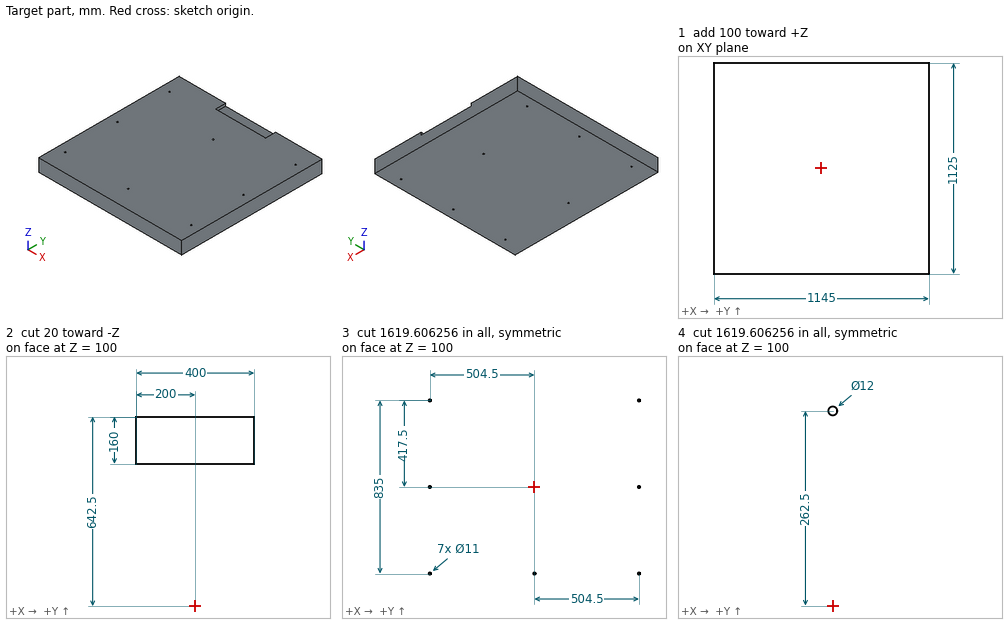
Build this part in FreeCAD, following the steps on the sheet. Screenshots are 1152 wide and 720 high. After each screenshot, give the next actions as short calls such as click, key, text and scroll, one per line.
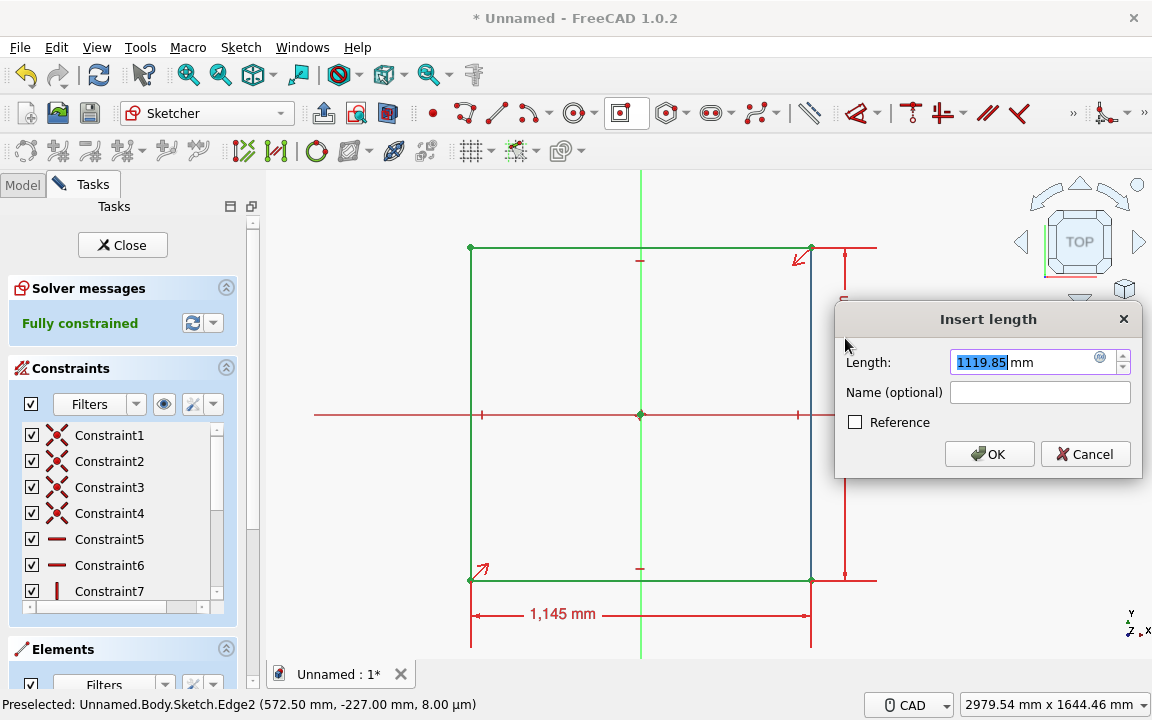
text(1125)
key(Return)
key(Escape)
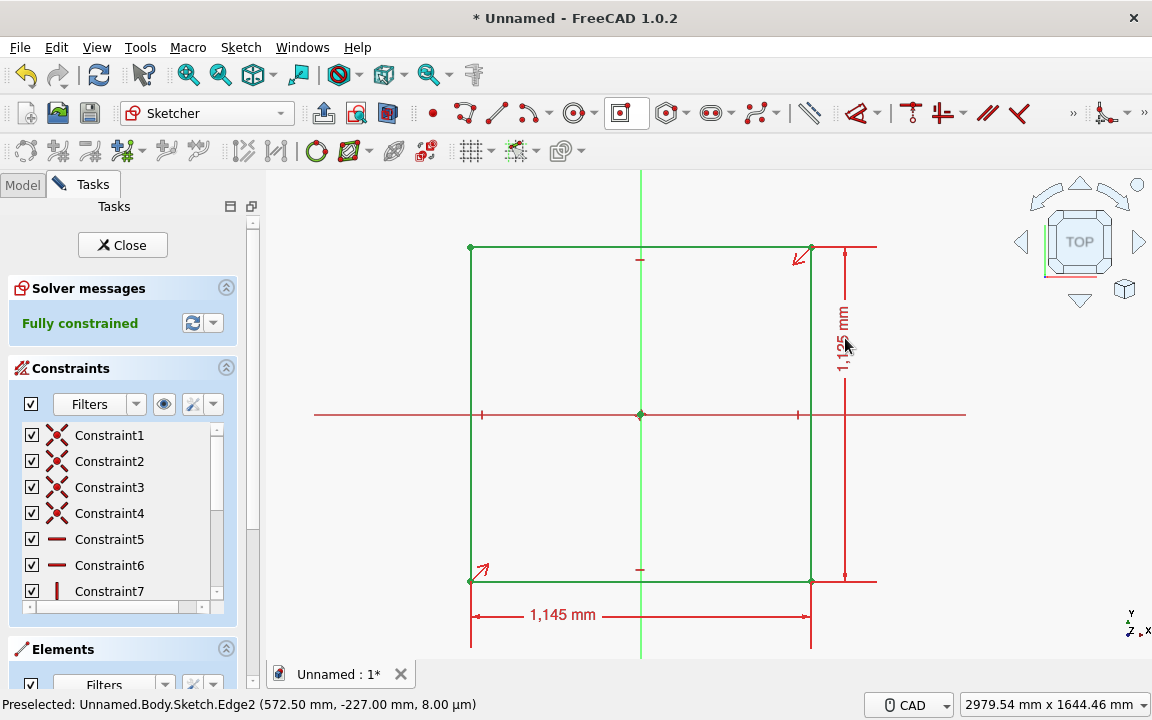
click(123, 245)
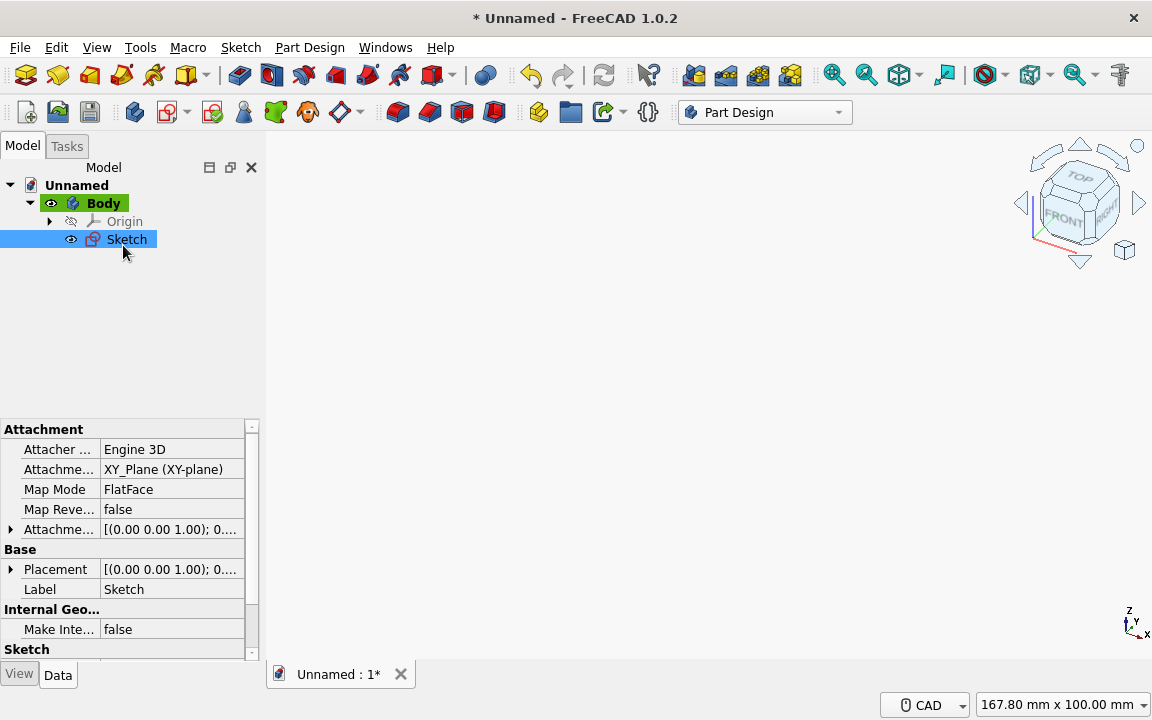
click(26, 76)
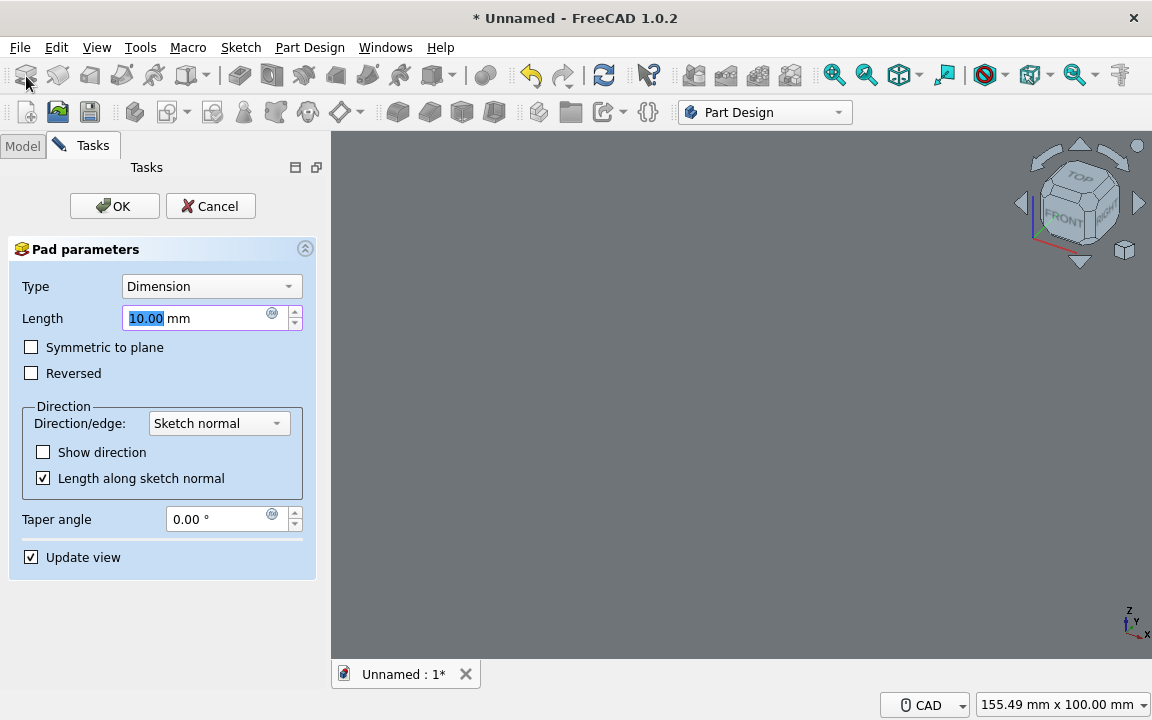
text(100)
key(Tab)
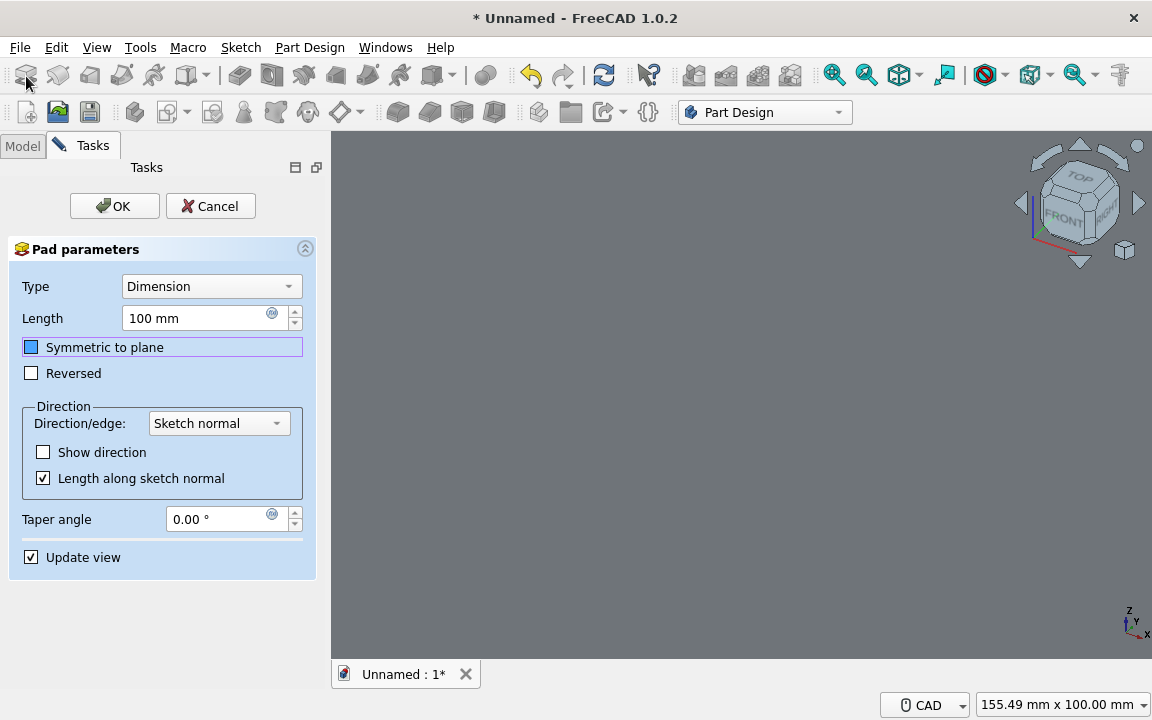
click(115, 206)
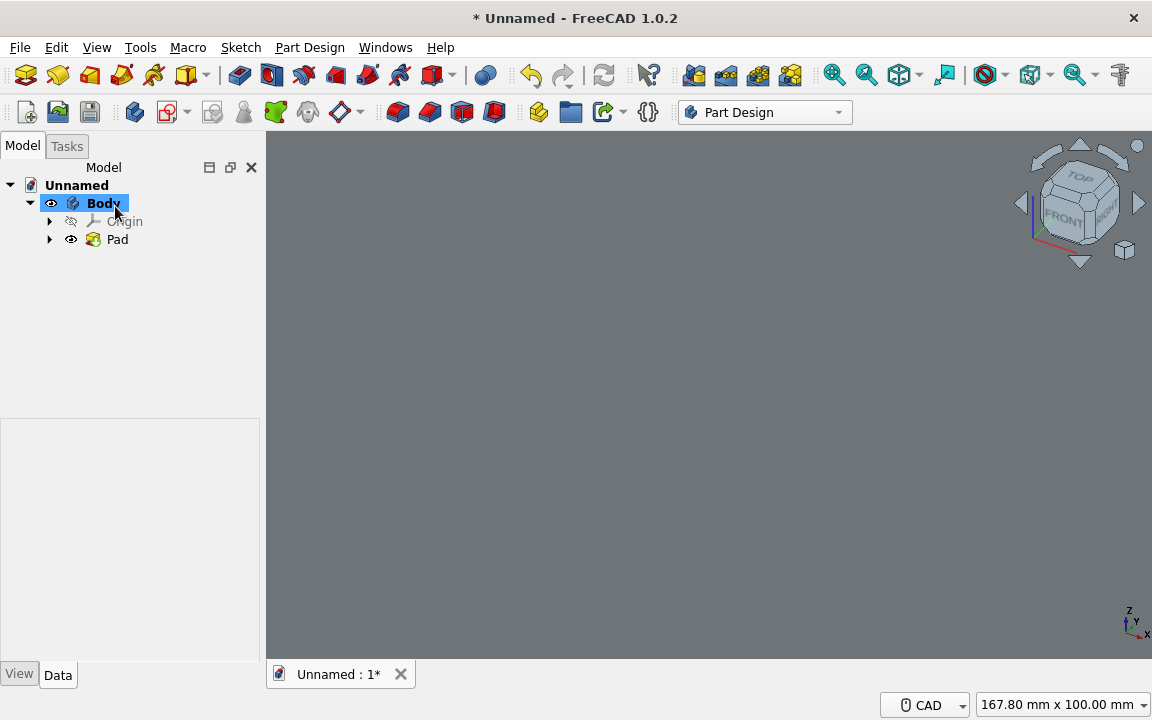
key(v)
key(f)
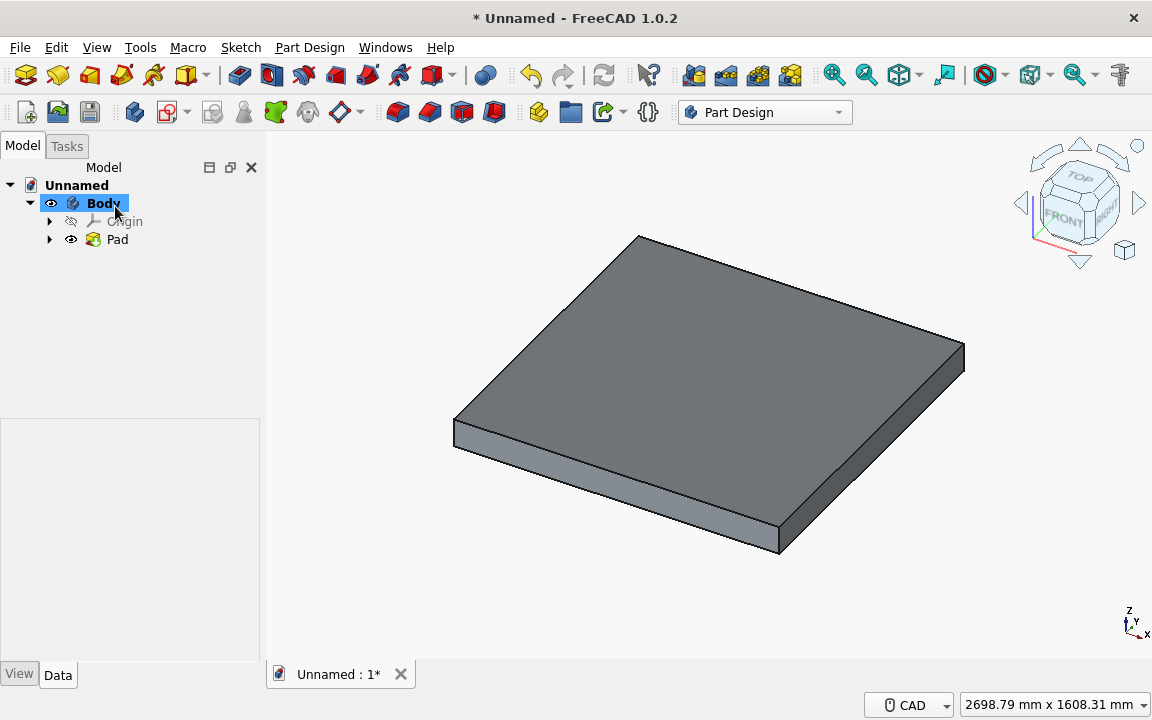
click(709, 381)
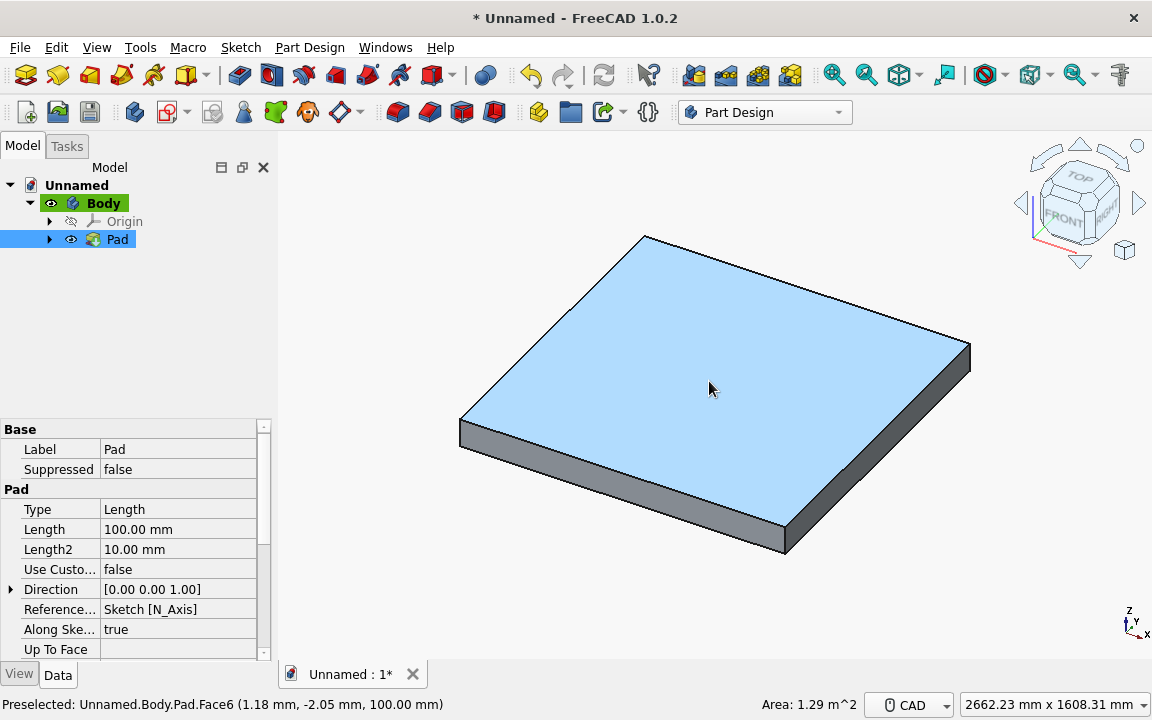
click(168, 112)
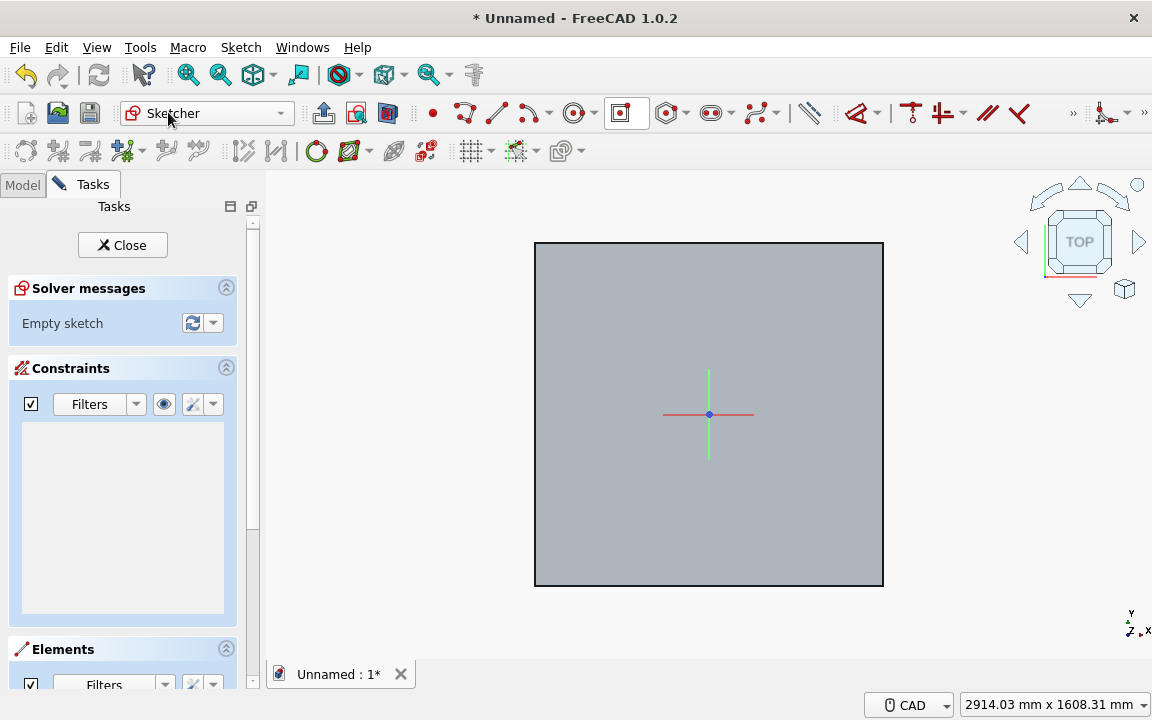
scroll(848, 198, up, 2)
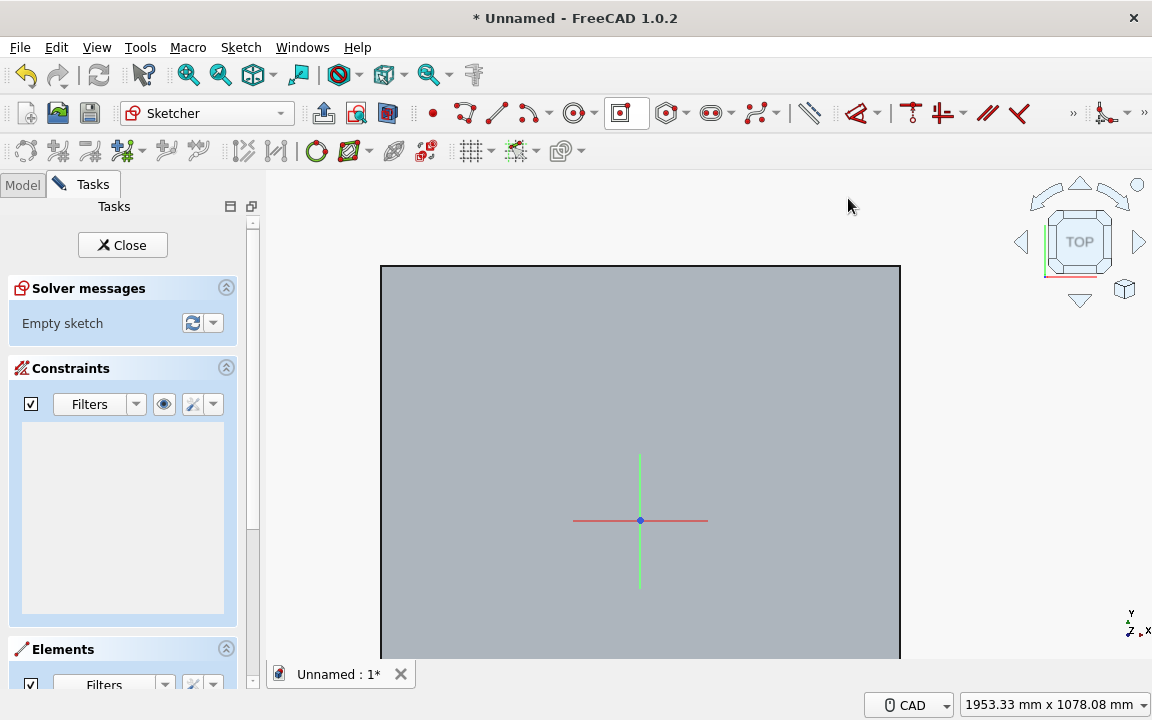
click(644, 114)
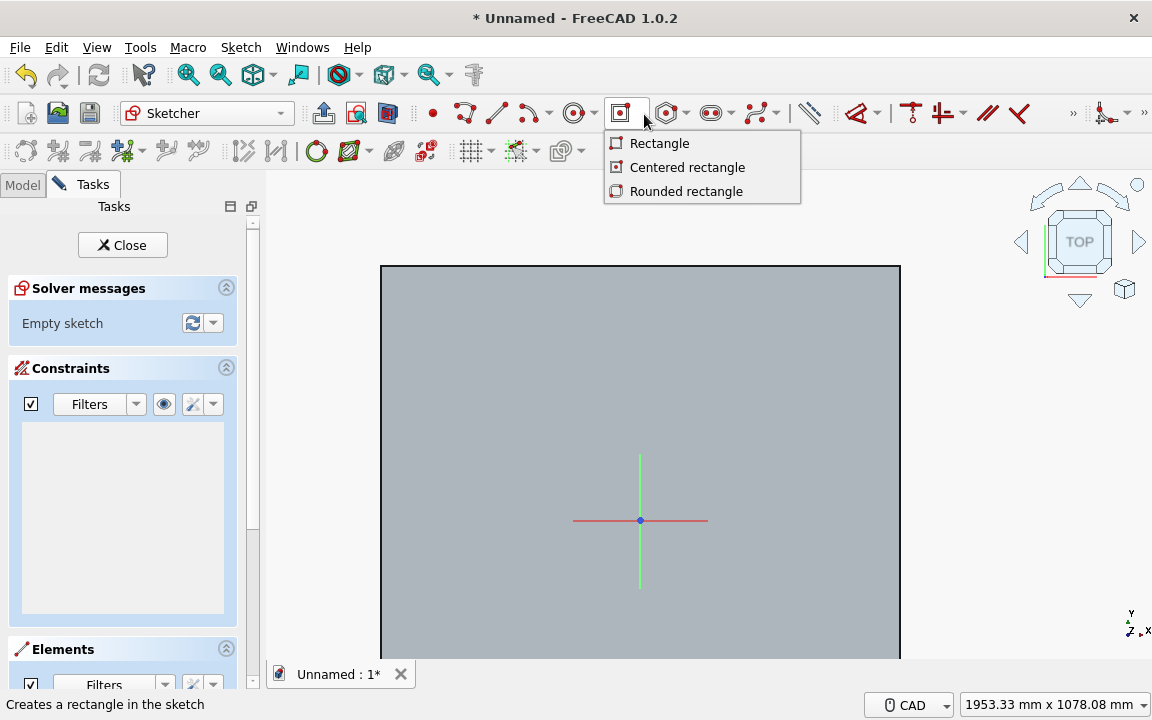
click(702, 143)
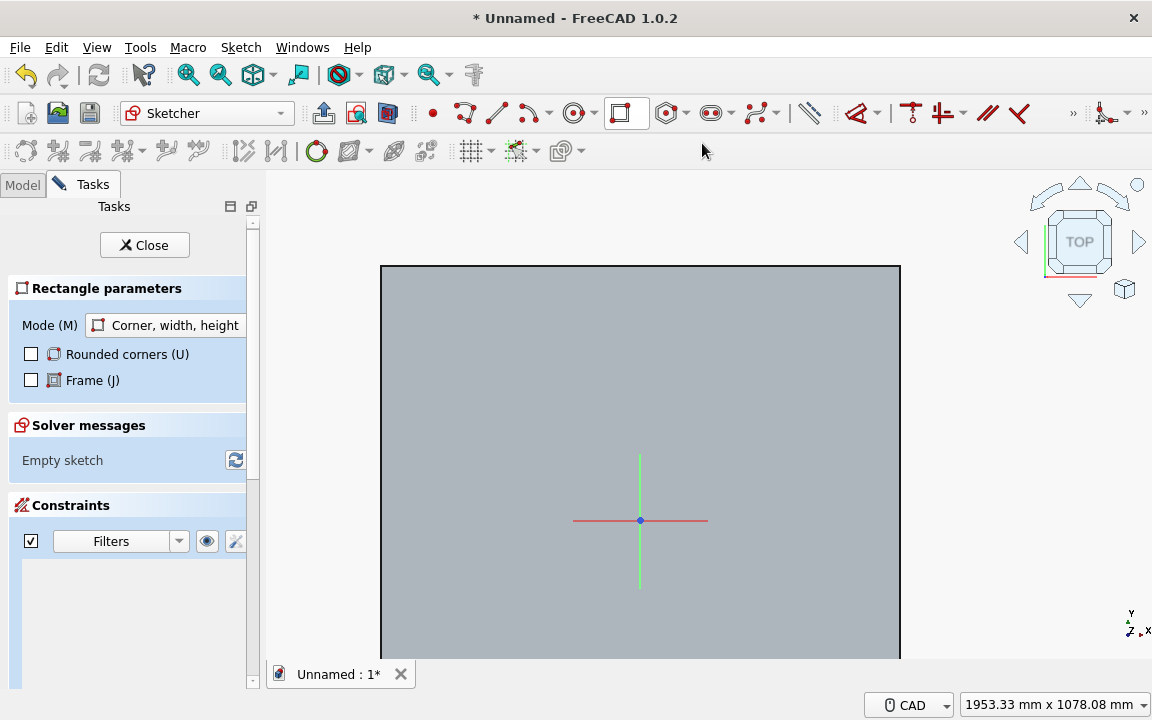
click(550, 230)
click(731, 302)
key(Escape)